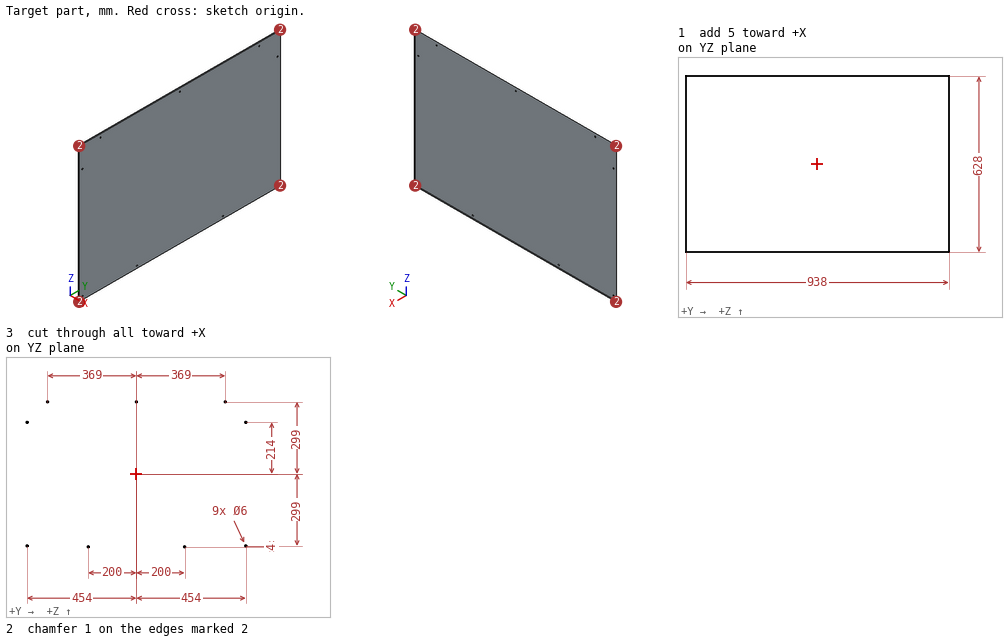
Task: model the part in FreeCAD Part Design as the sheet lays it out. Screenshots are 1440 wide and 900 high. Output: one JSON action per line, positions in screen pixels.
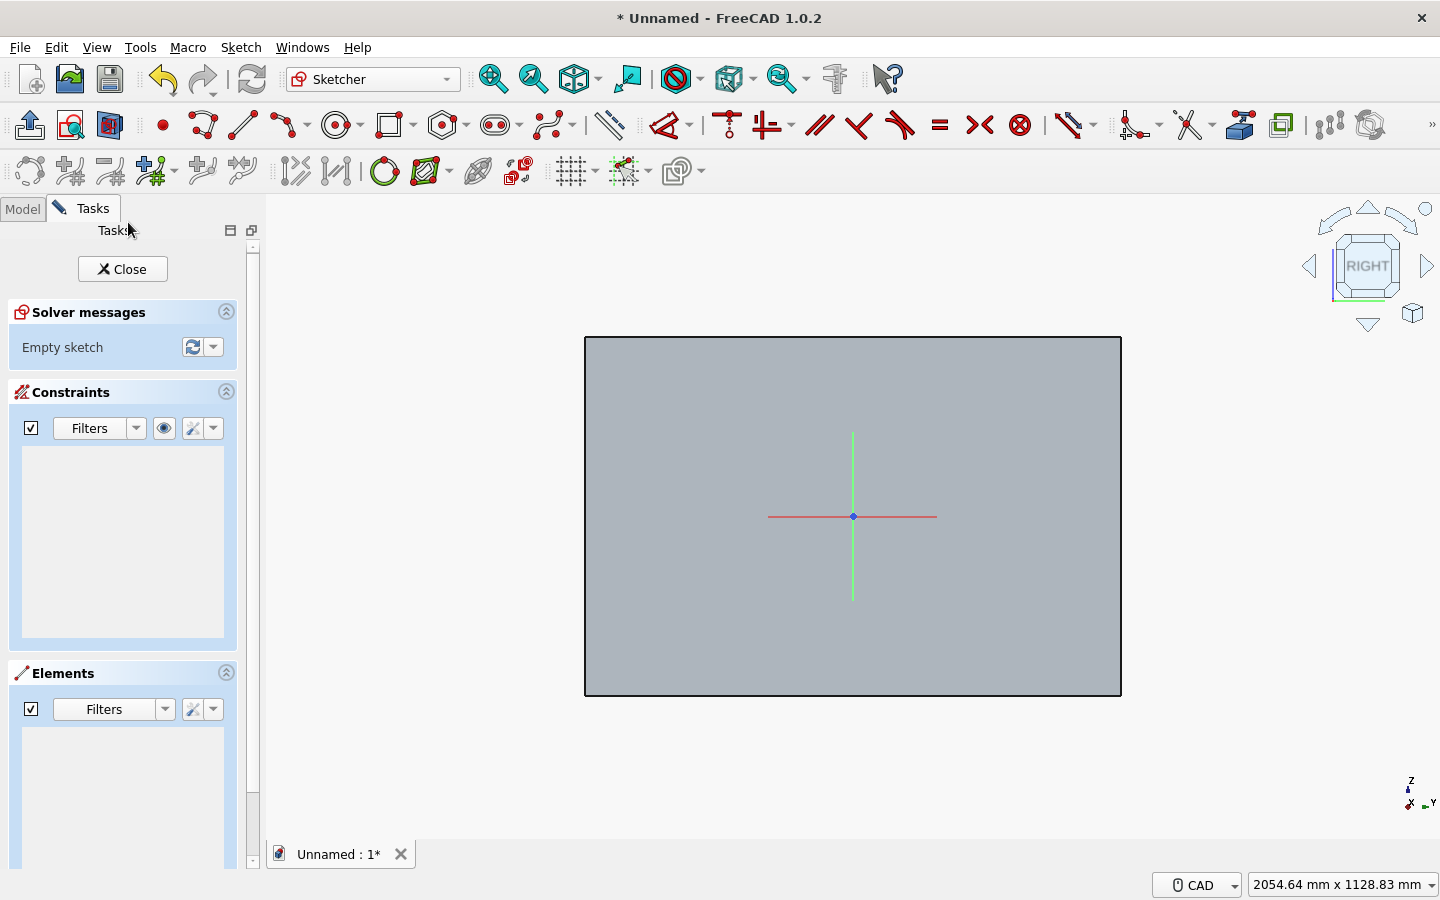
{"action": "key", "text": "g c"}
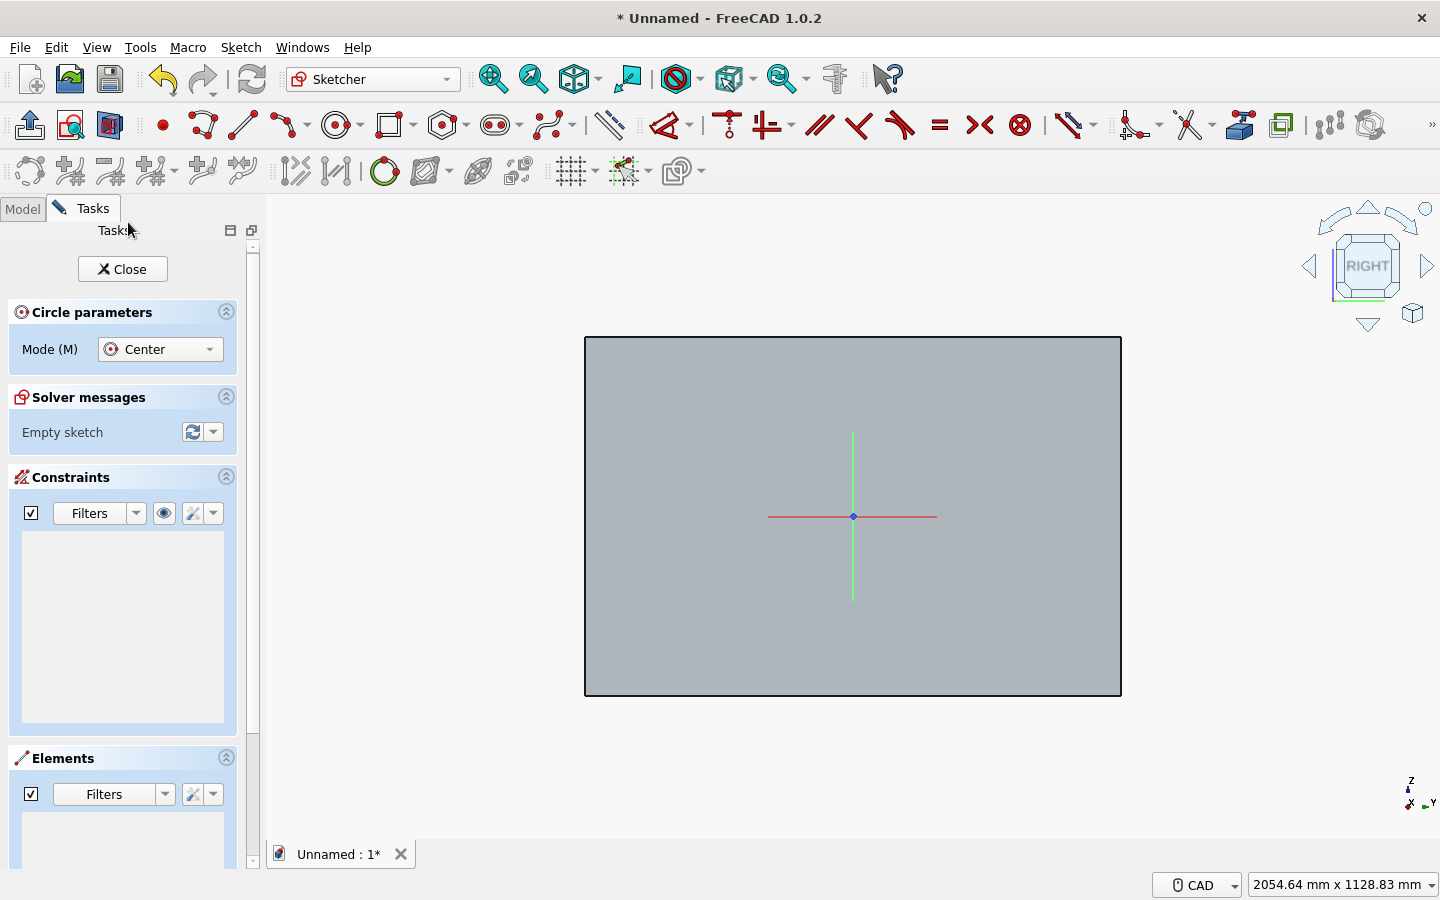
{"action": "scroll", "coordinate": [1112, 687], "scroll_direction": "up", "scroll_amount": 13}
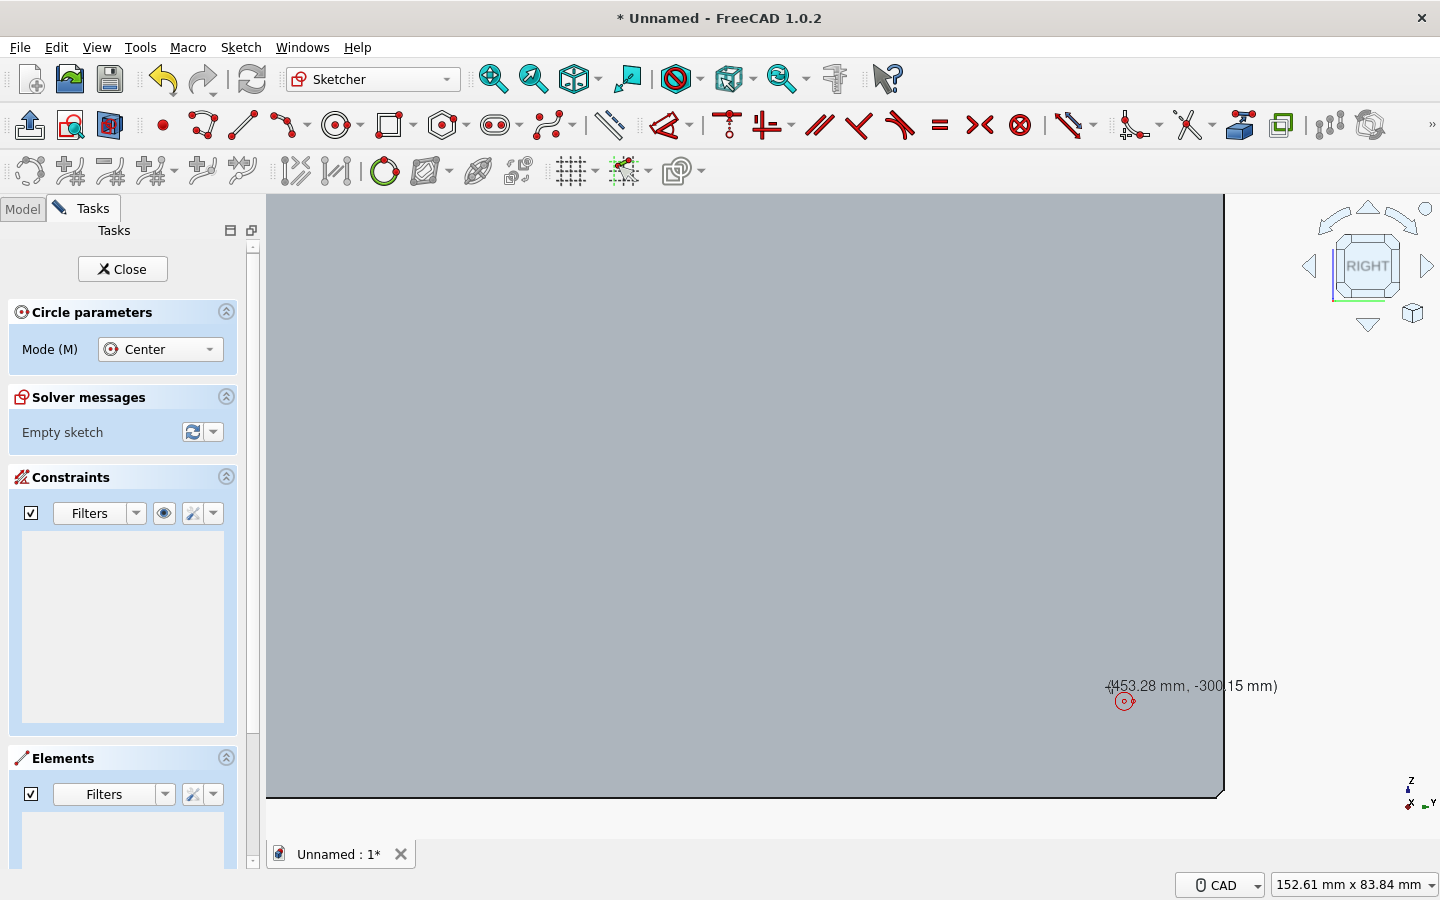
{"action": "scroll", "coordinate": [1101, 728], "scroll_direction": "down", "scroll_amount": 12}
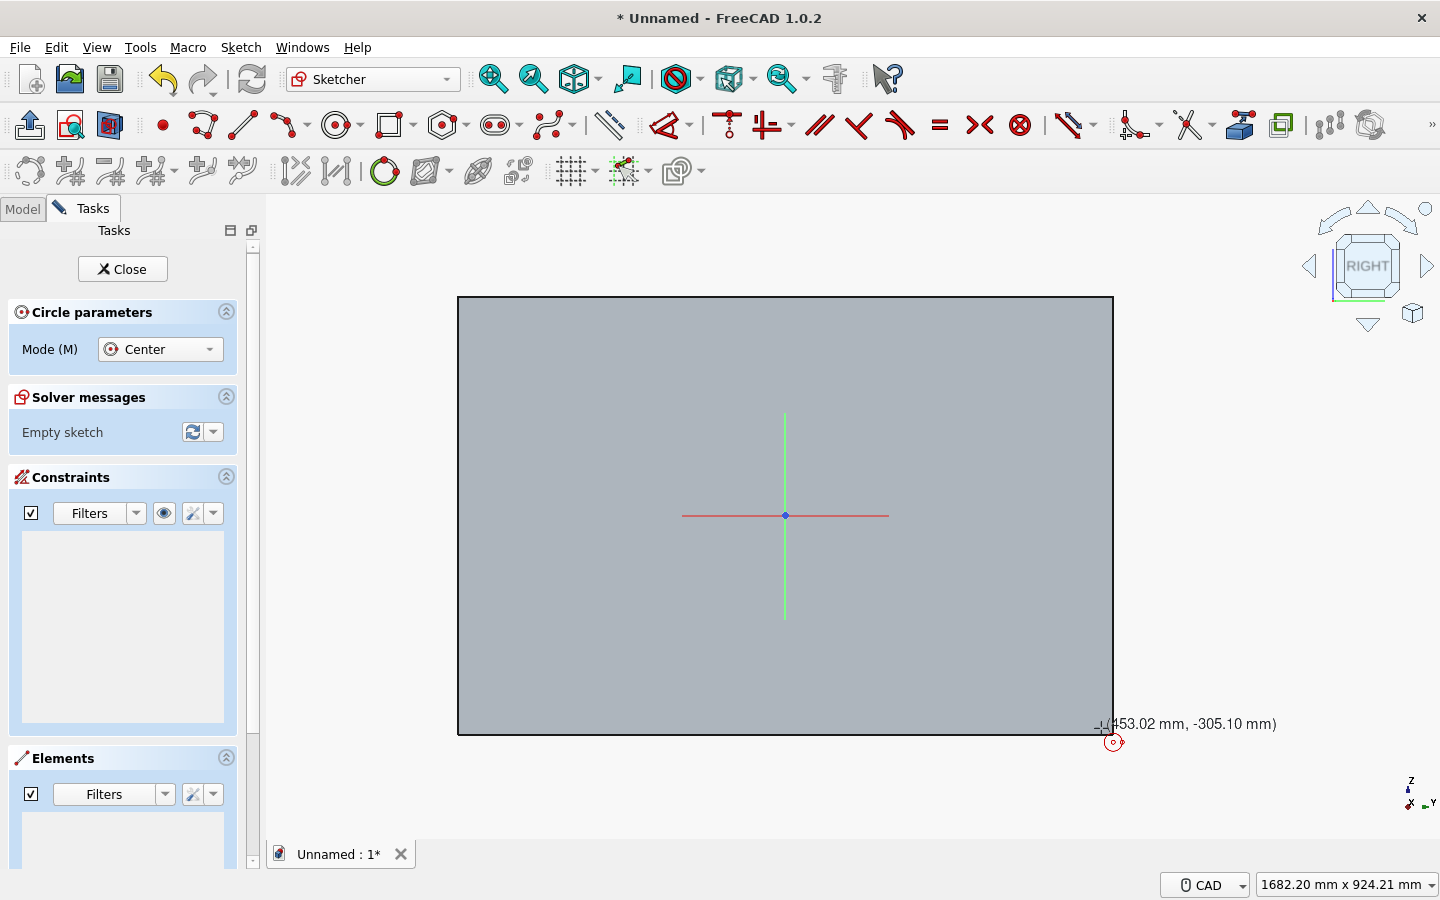
{"action": "left_click", "coordinate": [1102, 725]}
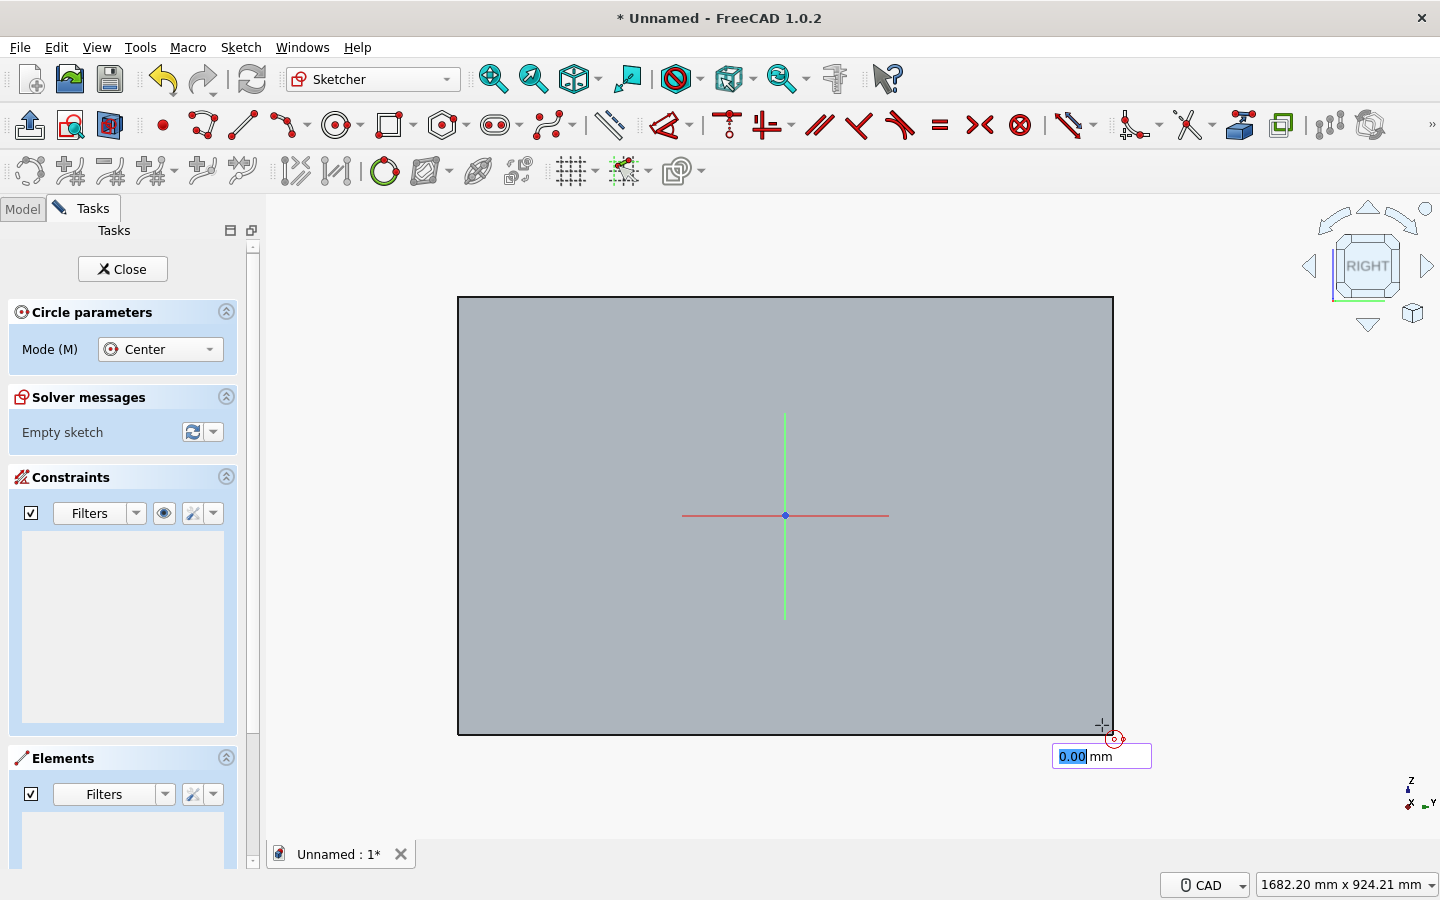
{"action": "scroll", "coordinate": [1104, 723], "scroll_direction": "up", "scroll_amount": 11}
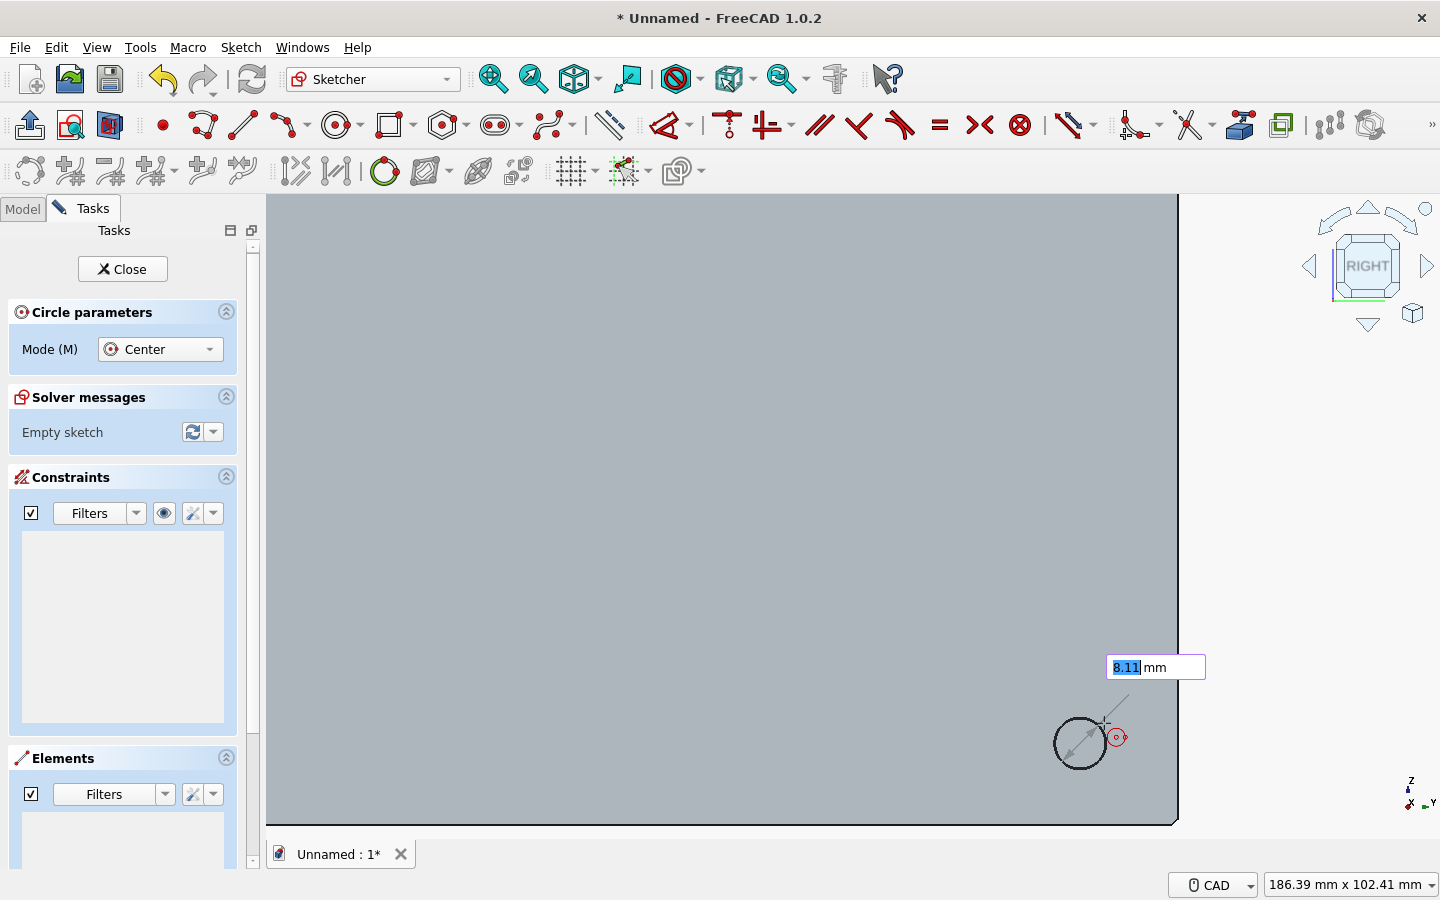
{"action": "left_click", "coordinate": [1097, 717]}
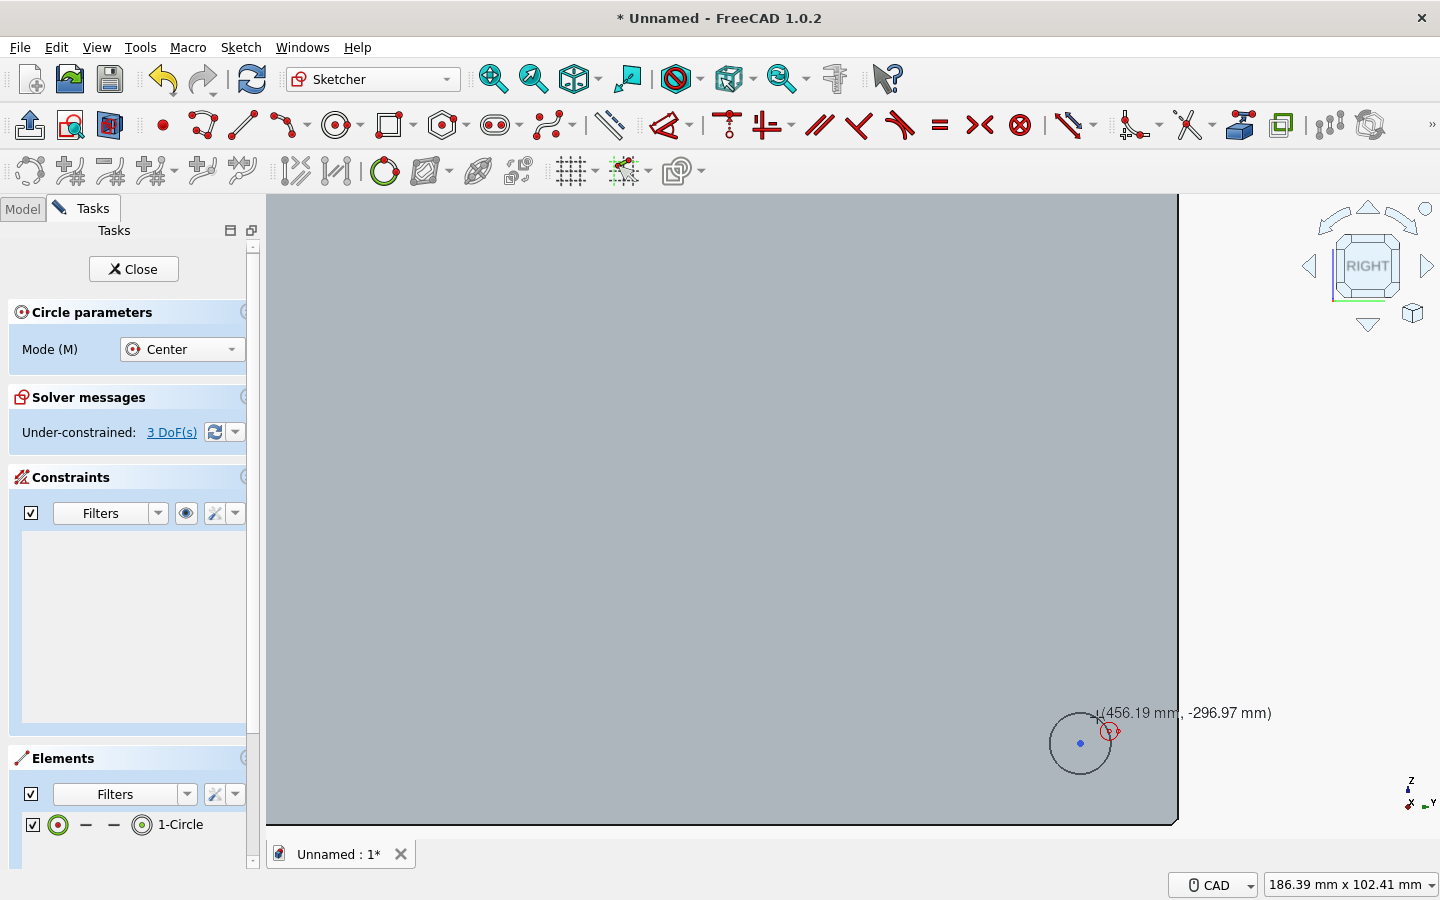
{"action": "scroll", "coordinate": [1104, 723], "scroll_direction": "down", "scroll_amount": 11}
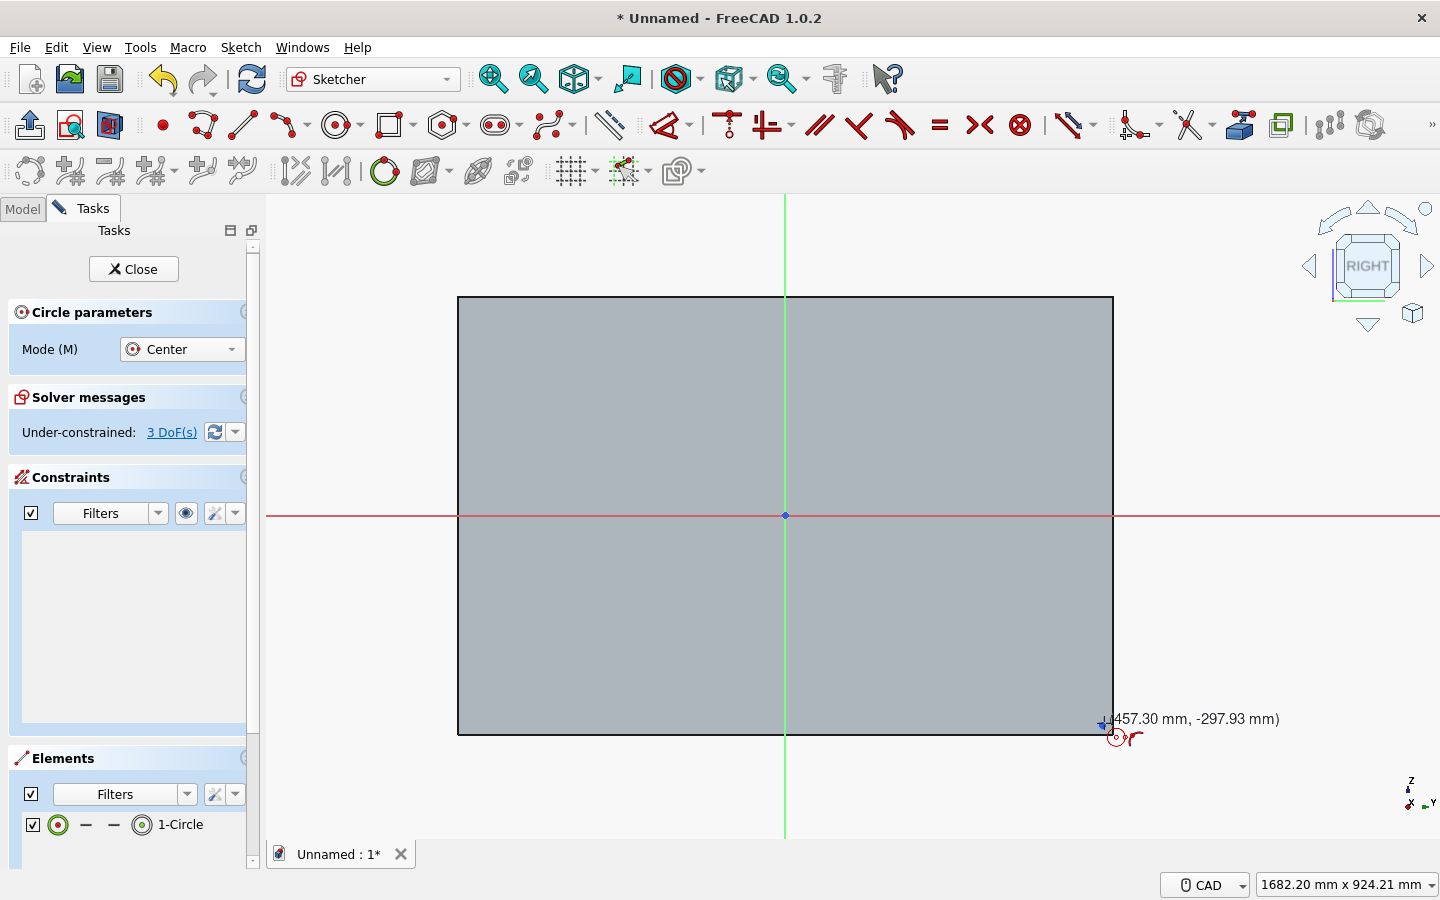
{"action": "scroll", "coordinate": [469, 725], "scroll_direction": "up", "scroll_amount": 12}